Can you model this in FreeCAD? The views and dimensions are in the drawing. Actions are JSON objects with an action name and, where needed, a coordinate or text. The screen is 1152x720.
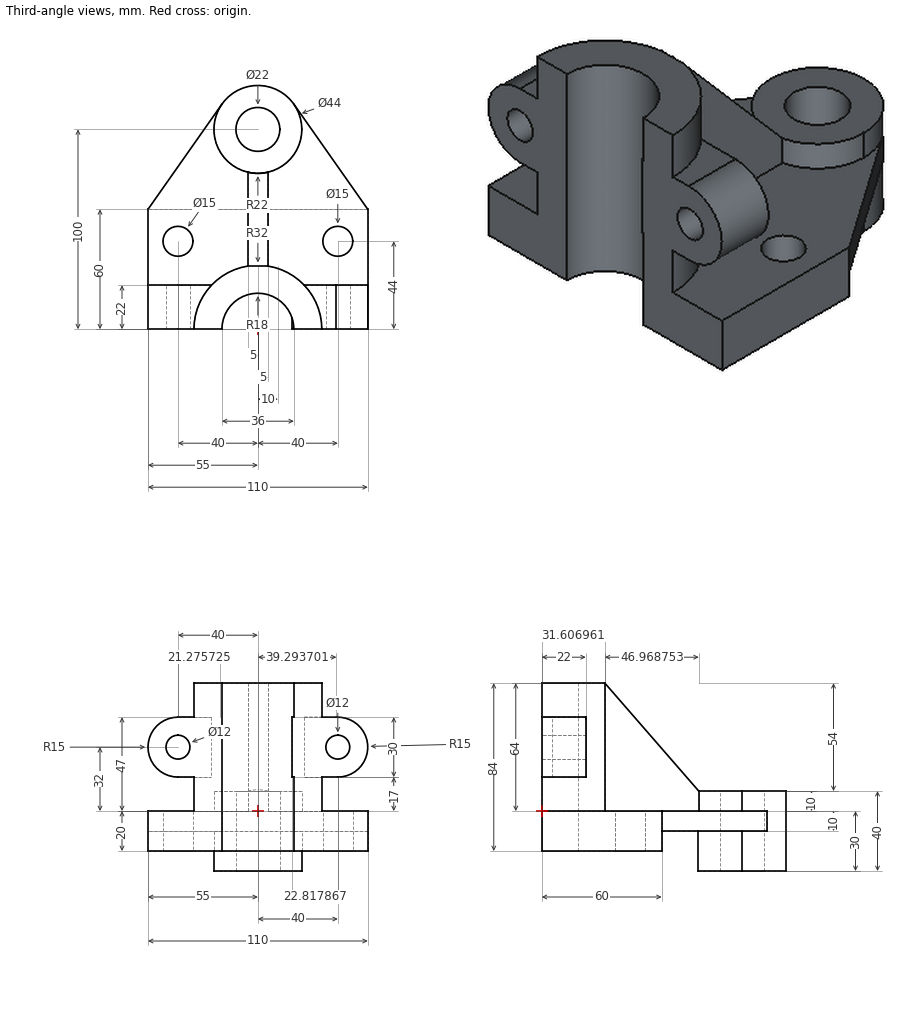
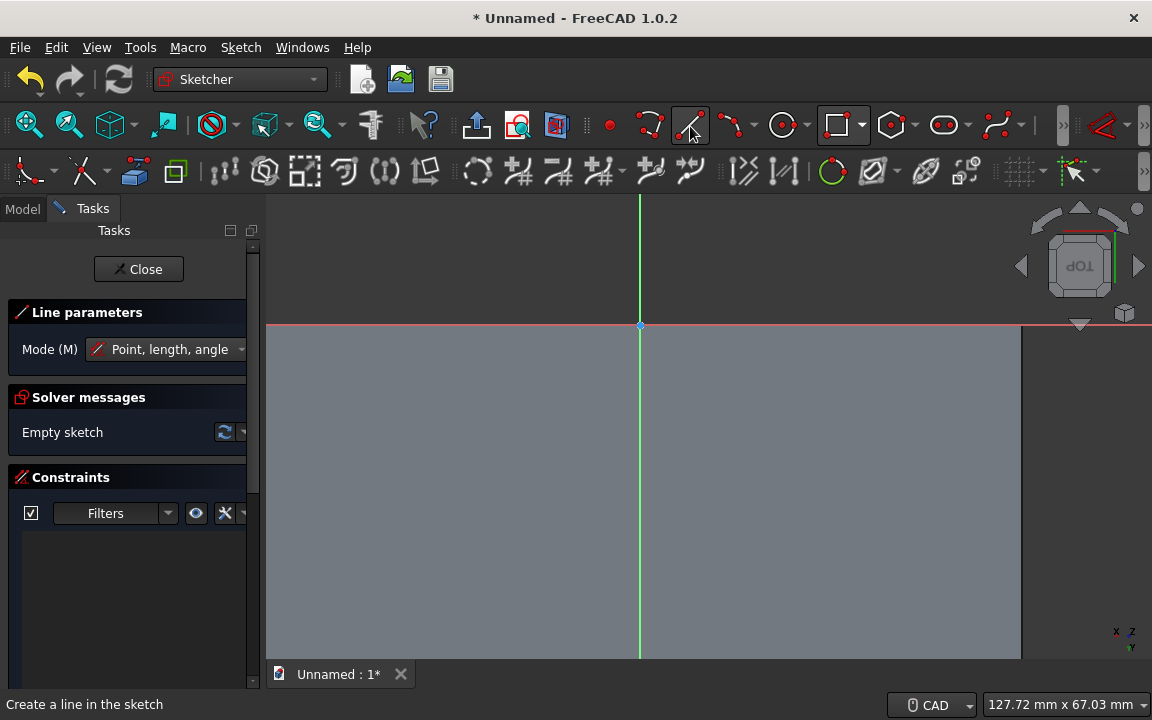
{"action": "left_click", "coordinate": [862, 325]}
{"action": "left_click", "coordinate": [418, 334]}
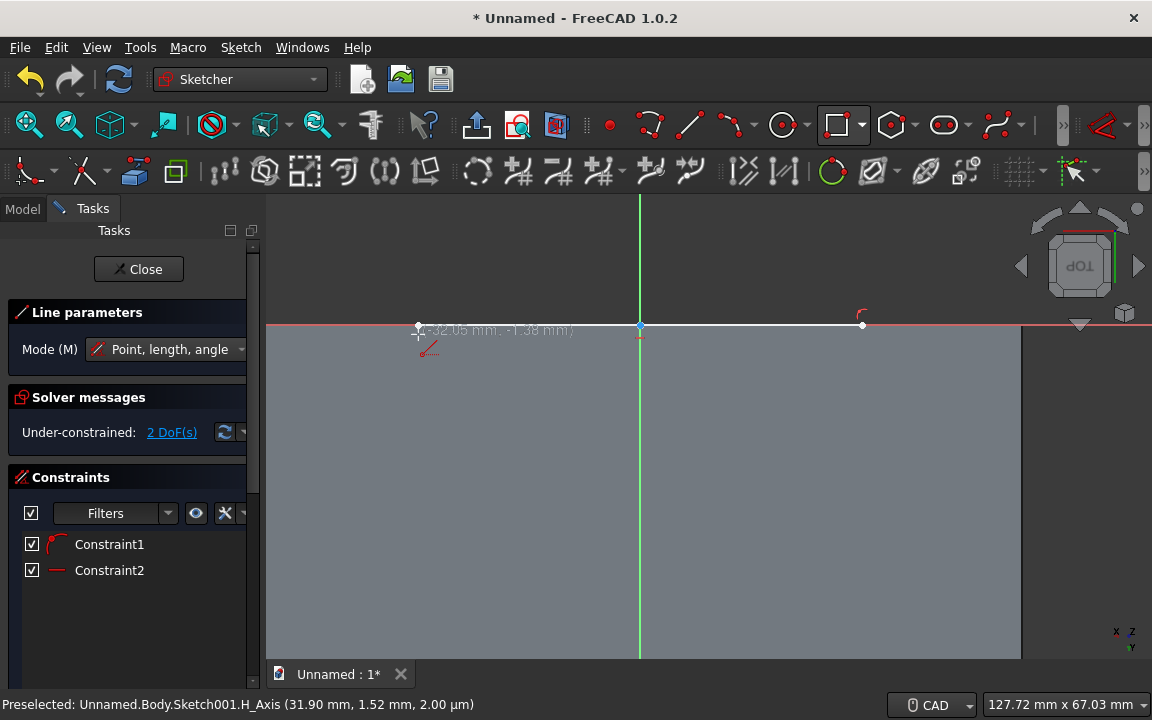
{"action": "left_click", "coordinate": [730, 126]}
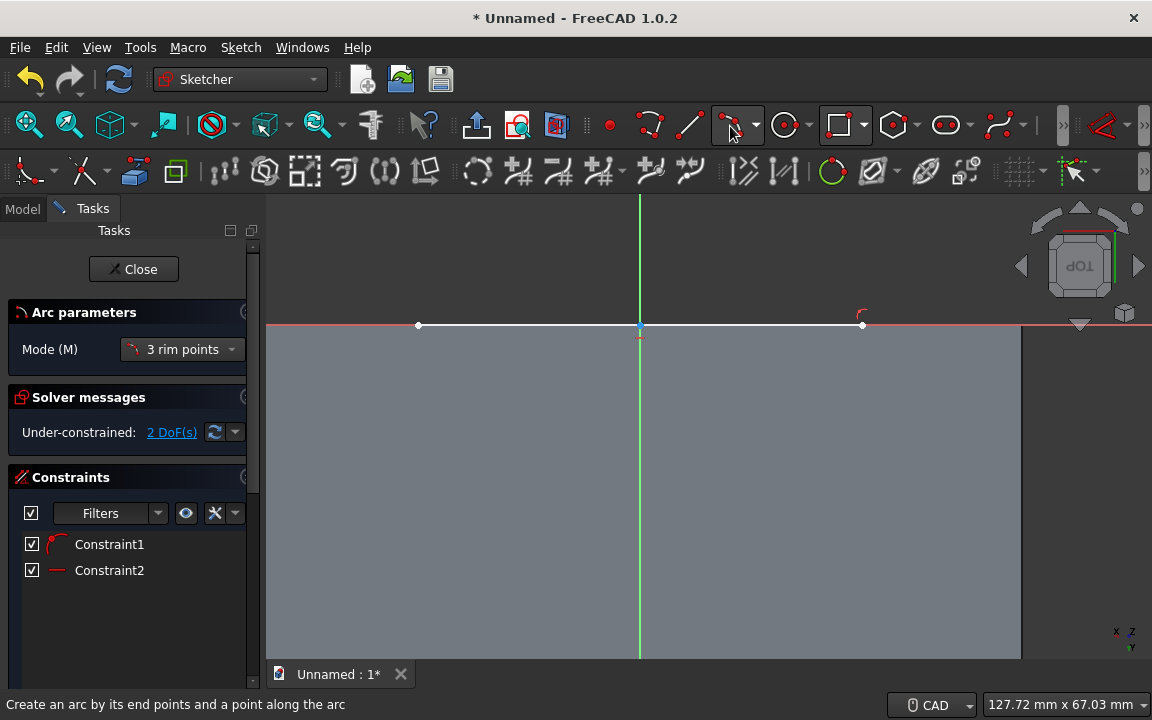
{"action": "left_click", "coordinate": [418, 325]}
{"action": "left_click", "coordinate": [862, 325]}
{"action": "left_click", "coordinate": [572, 537]}
{"action": "key", "text": "Escape"}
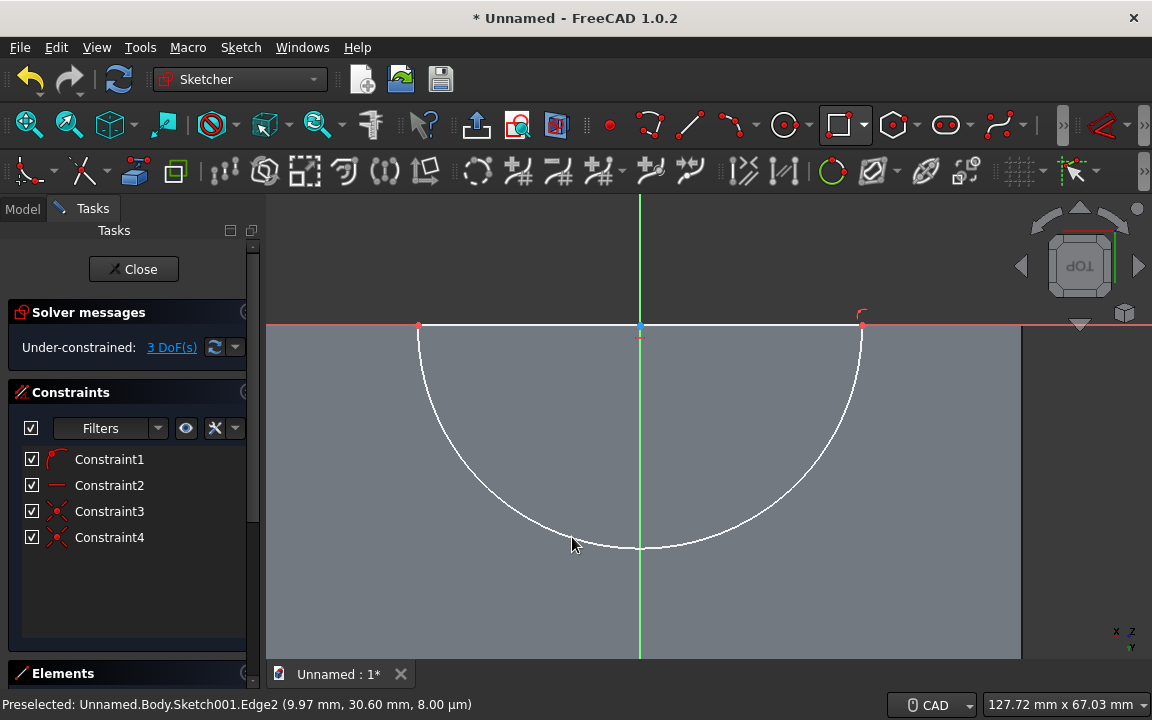
{"action": "left_click_drag", "start_coordinate": [630, 315], "coordinate": [650, 337]}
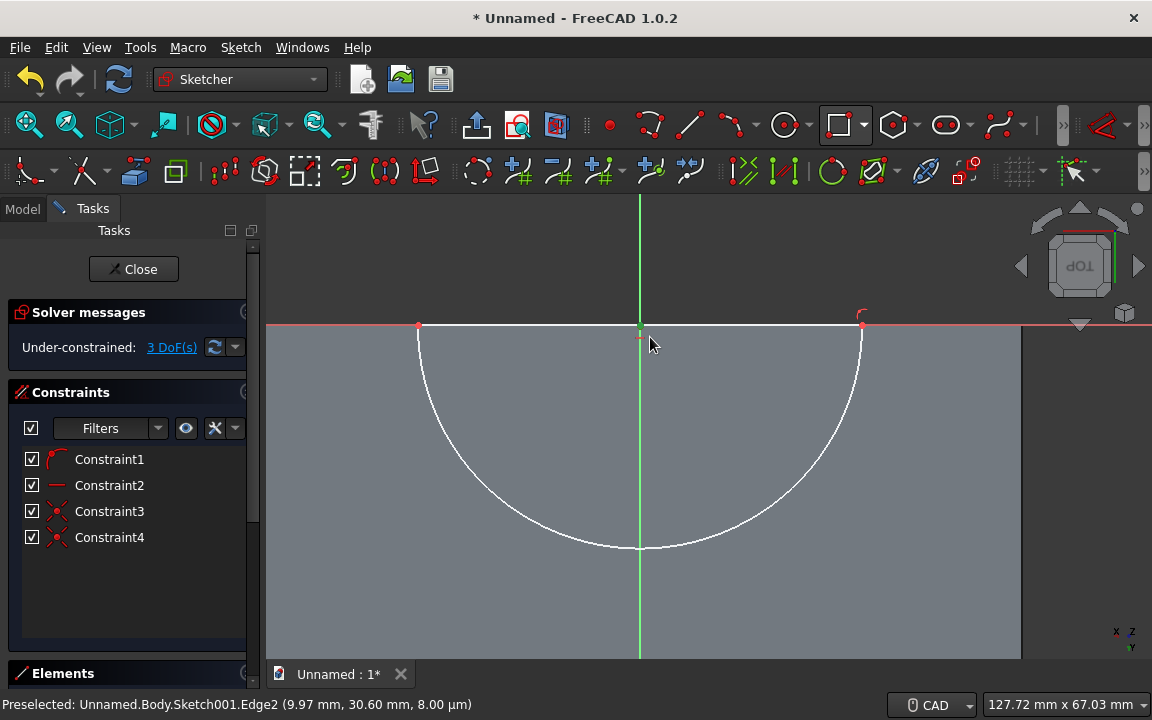
{"action": "key", "text": "c"}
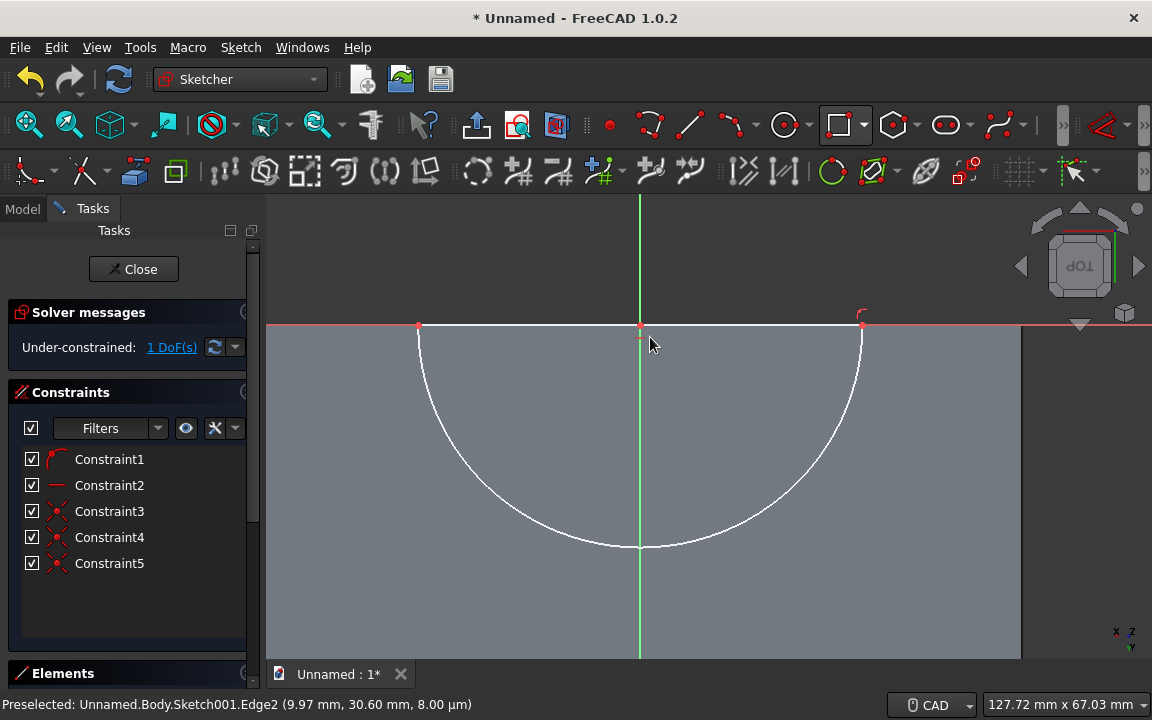
{"action": "left_click", "coordinate": [1102, 126]}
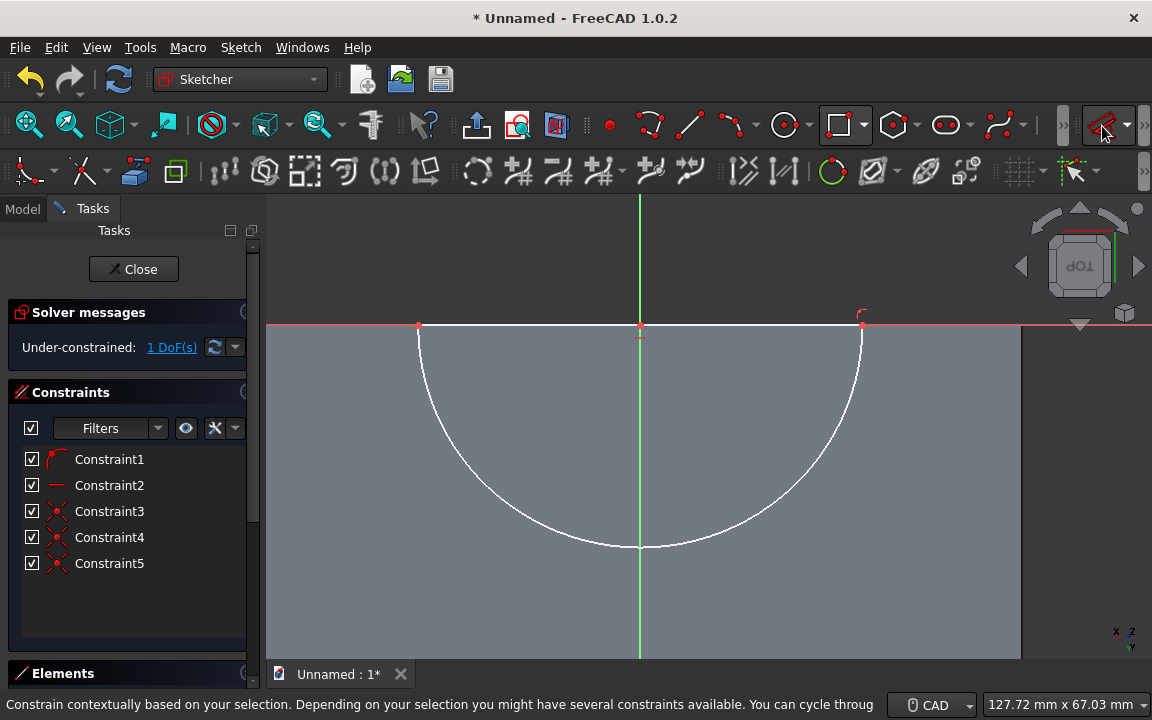
{"action": "left_click", "coordinate": [510, 505]}
{"action": "left_click", "coordinate": [491, 531]}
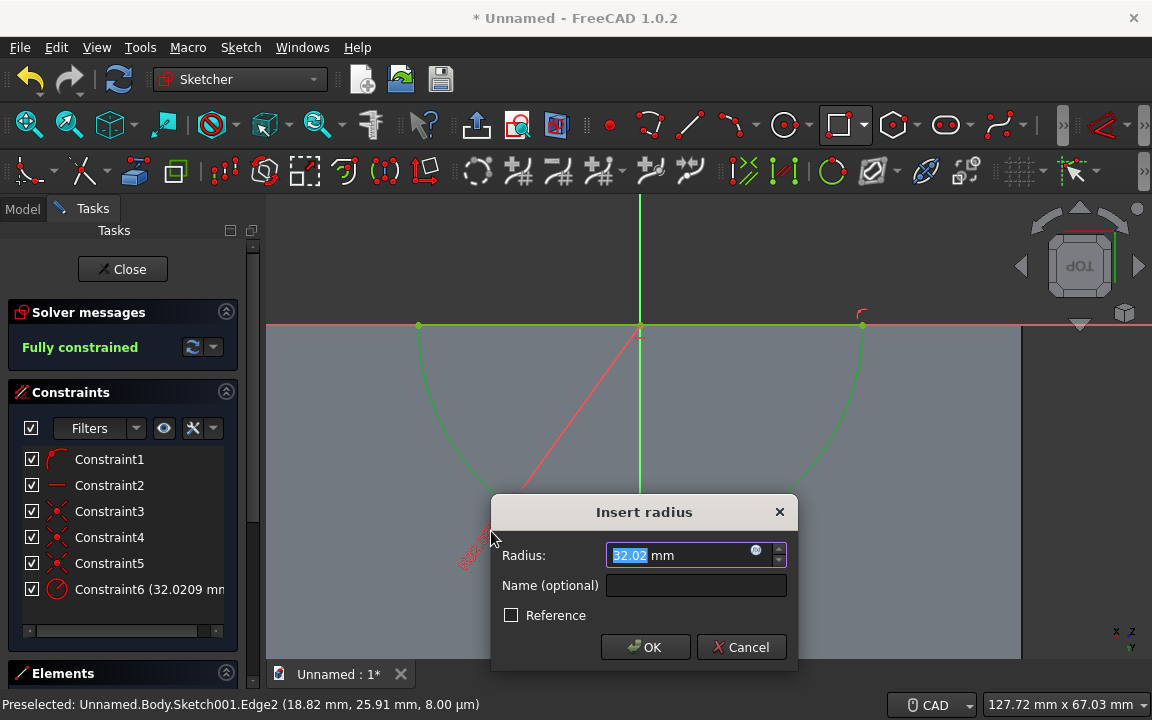
{"action": "type", "text": "32"}
{"action": "key", "text": "Return"}
{"action": "key", "text": "Escape"}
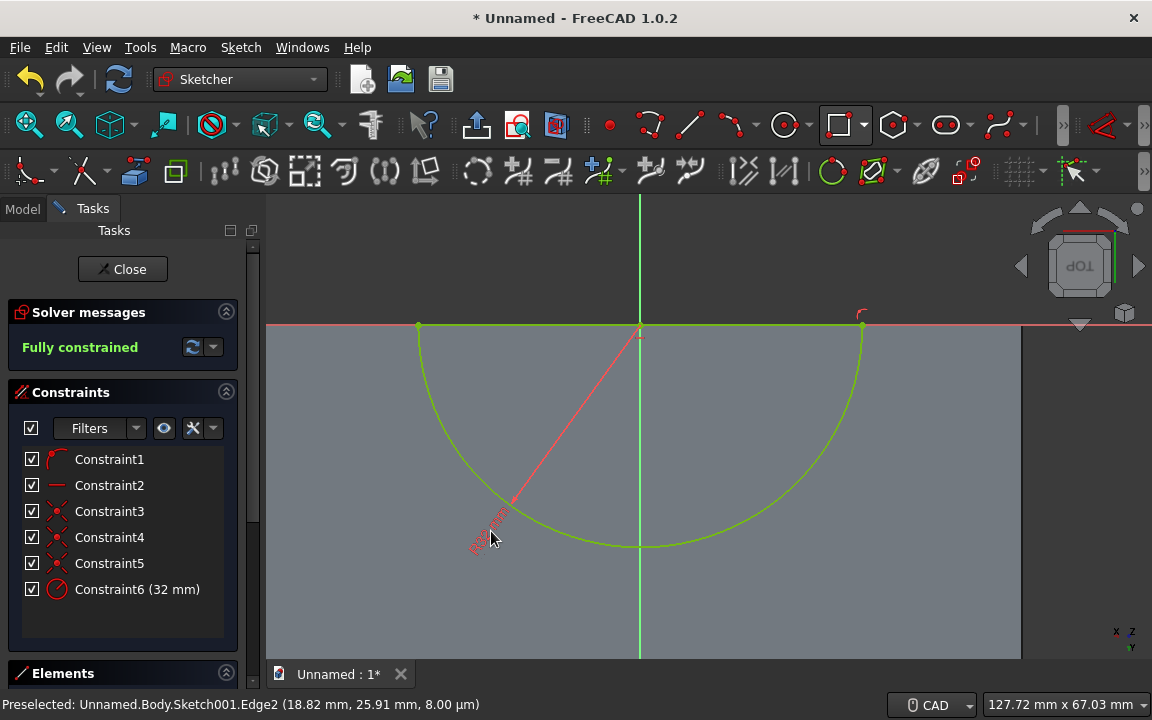
{"action": "left_click", "coordinate": [123, 269]}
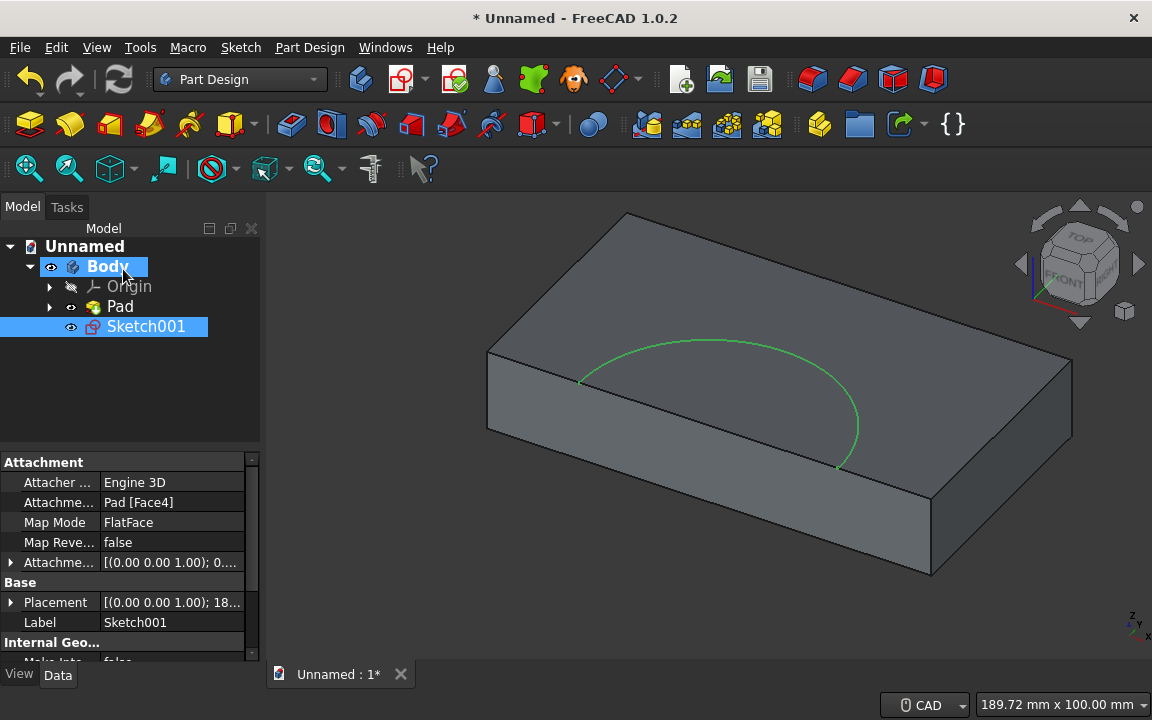
{"action": "left_click", "coordinate": [30, 124]}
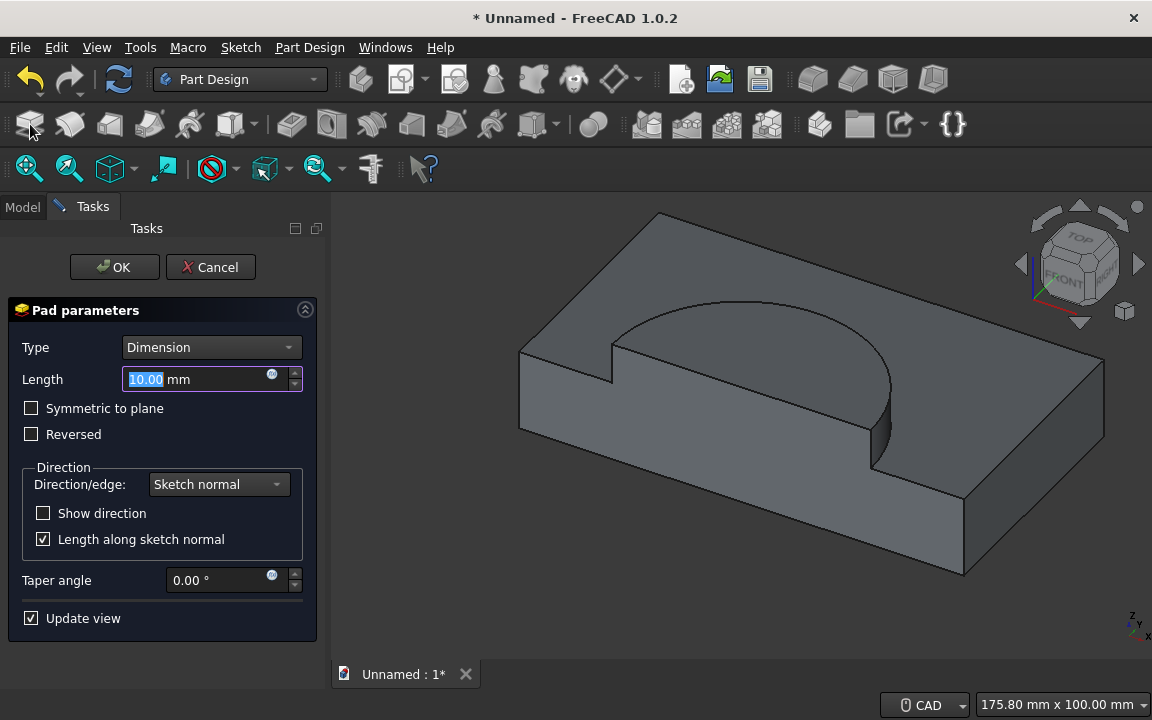
{"action": "type", "text": "64"}
{"action": "key", "text": "Tab"}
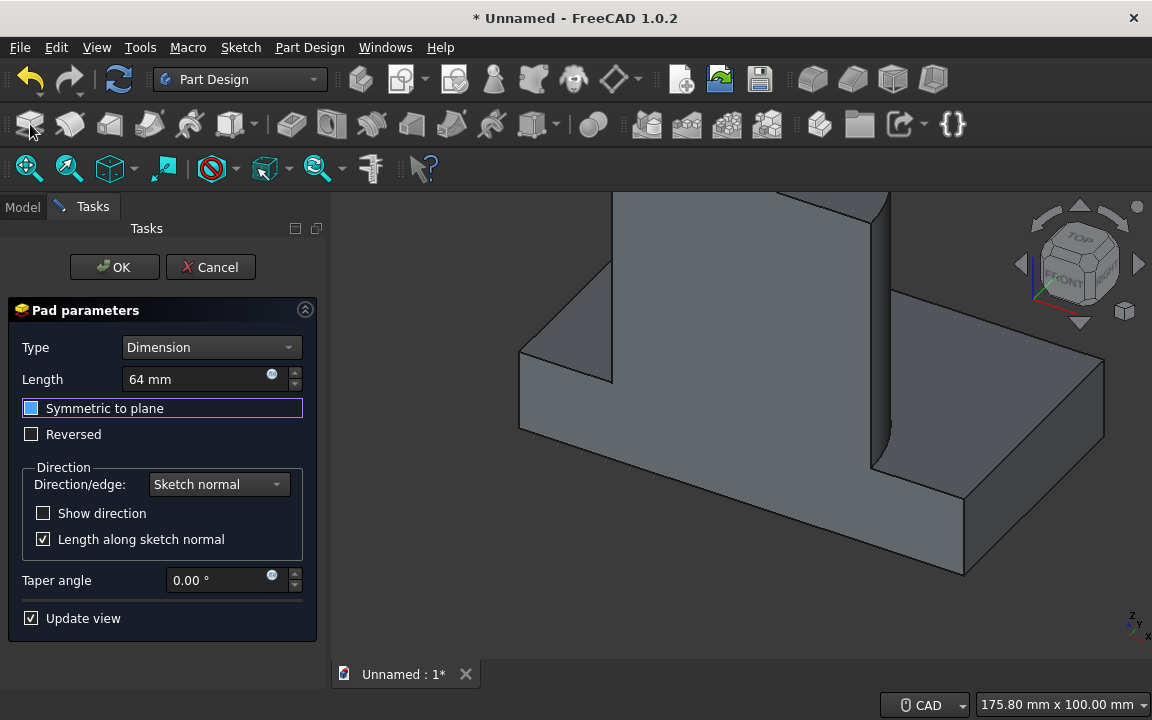
{"action": "left_click", "coordinate": [115, 267]}